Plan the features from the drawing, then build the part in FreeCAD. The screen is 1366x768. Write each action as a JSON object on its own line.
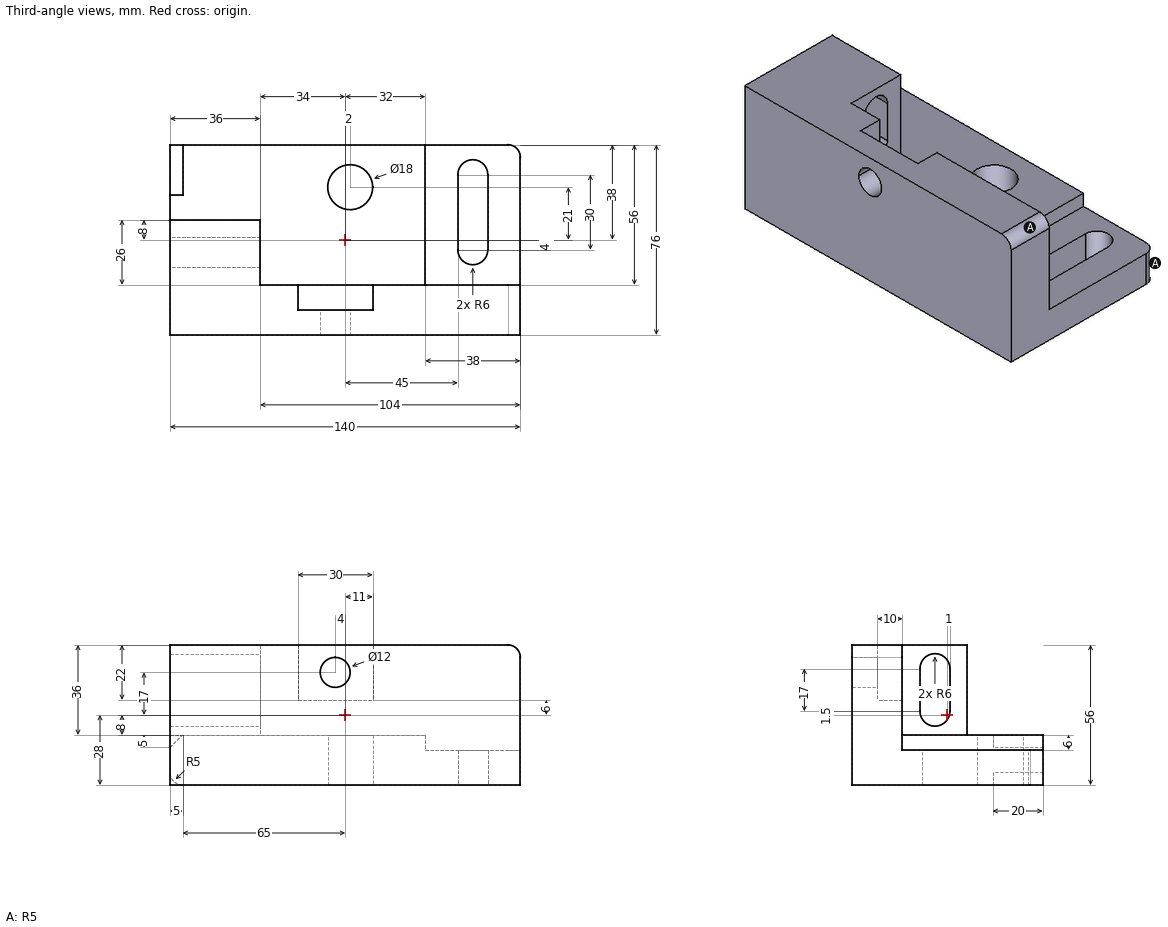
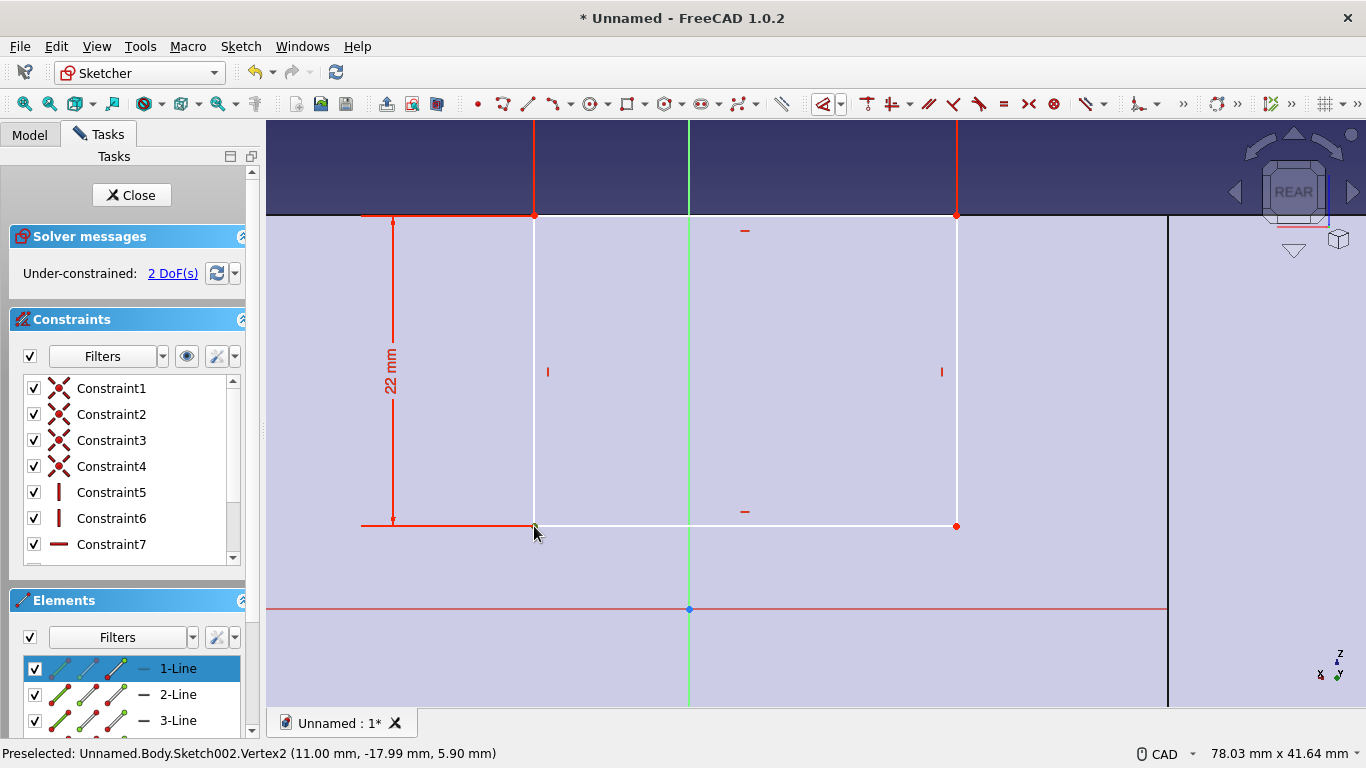
{"action": "key", "text": "i"}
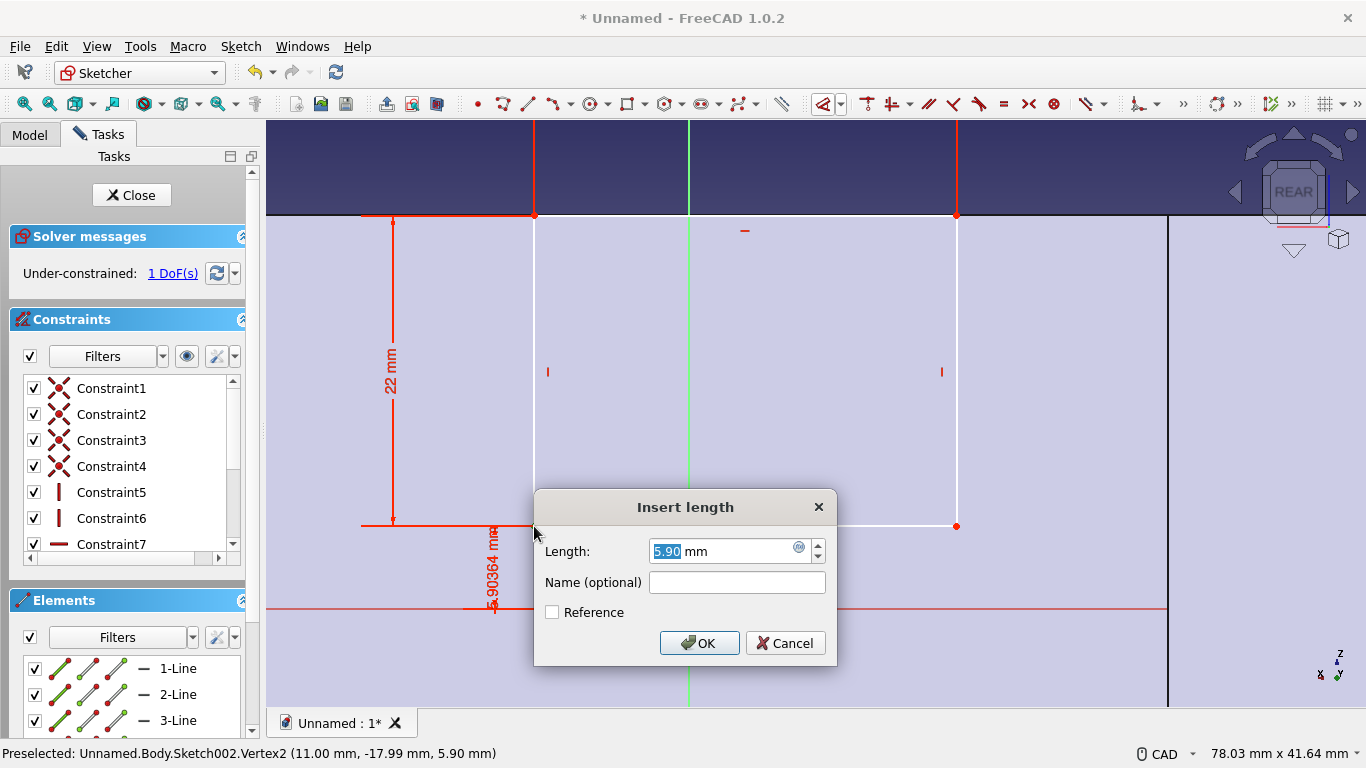
{"action": "type", "text": "6"}
{"action": "key", "text": "Return"}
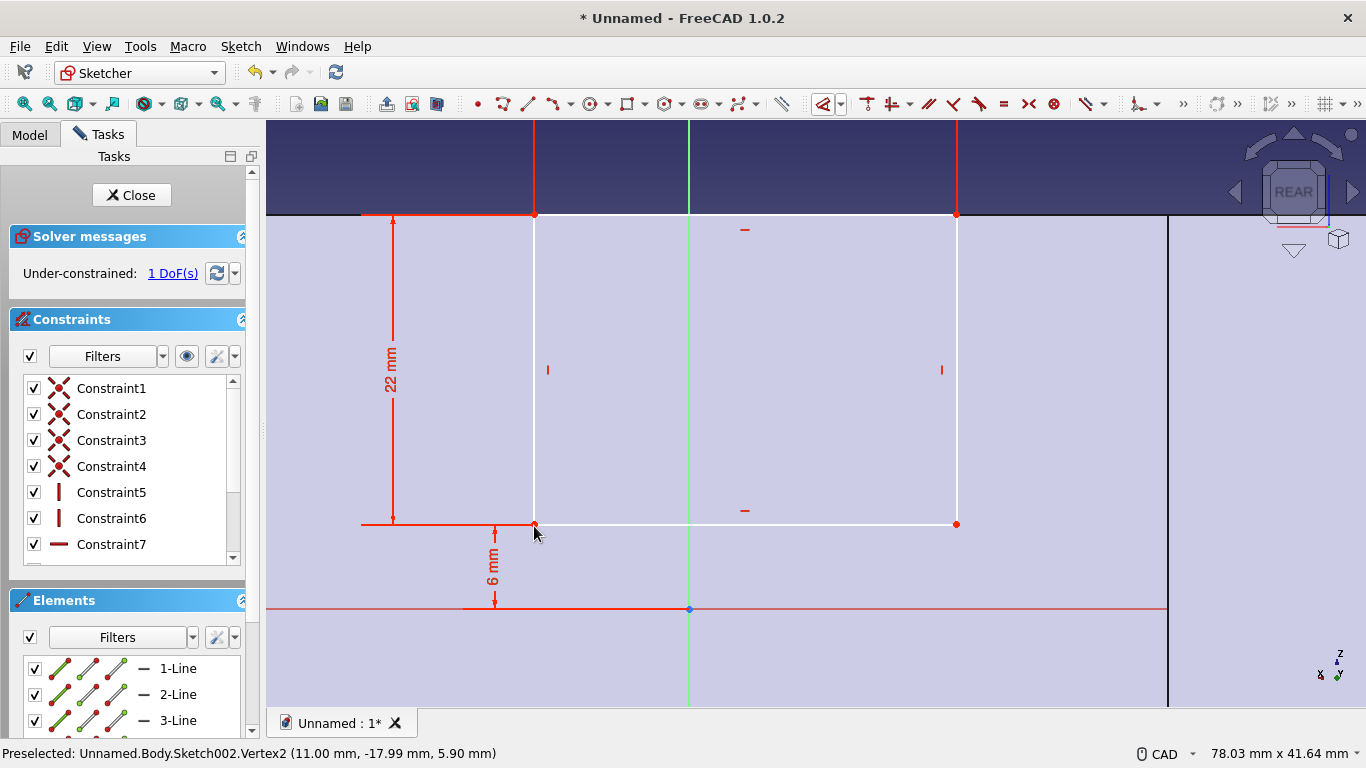
{"action": "left_click", "coordinate": [534, 215]}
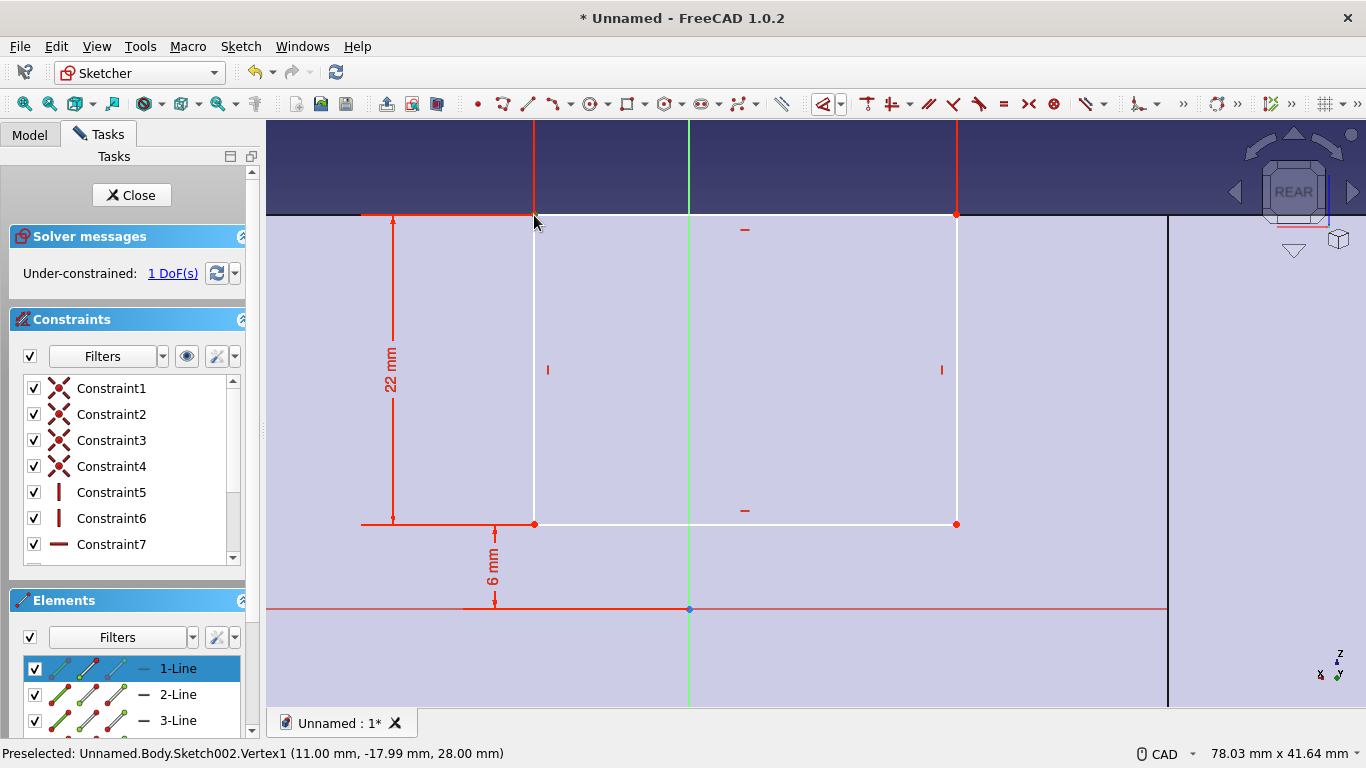
{"action": "key", "text": "l"}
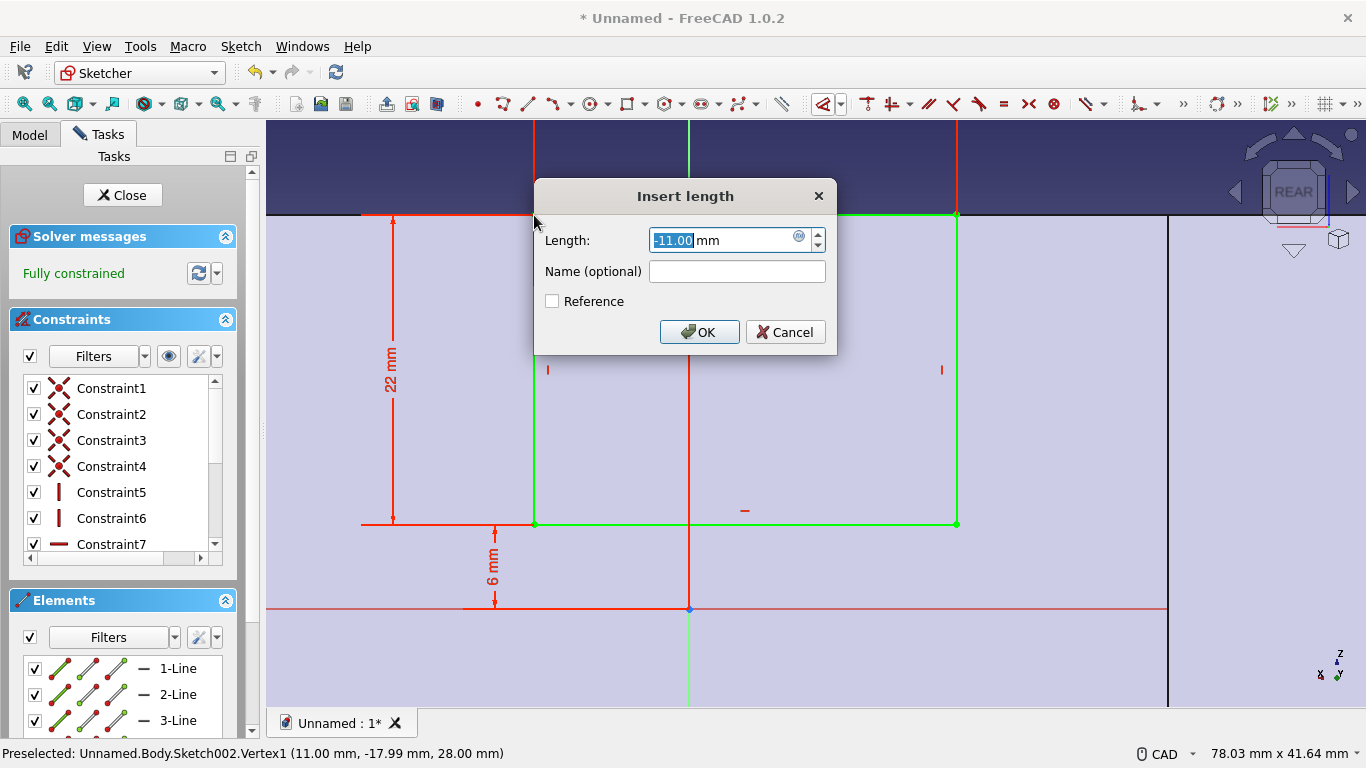
{"action": "type", "text": "-11"}
{"action": "key", "text": "Return"}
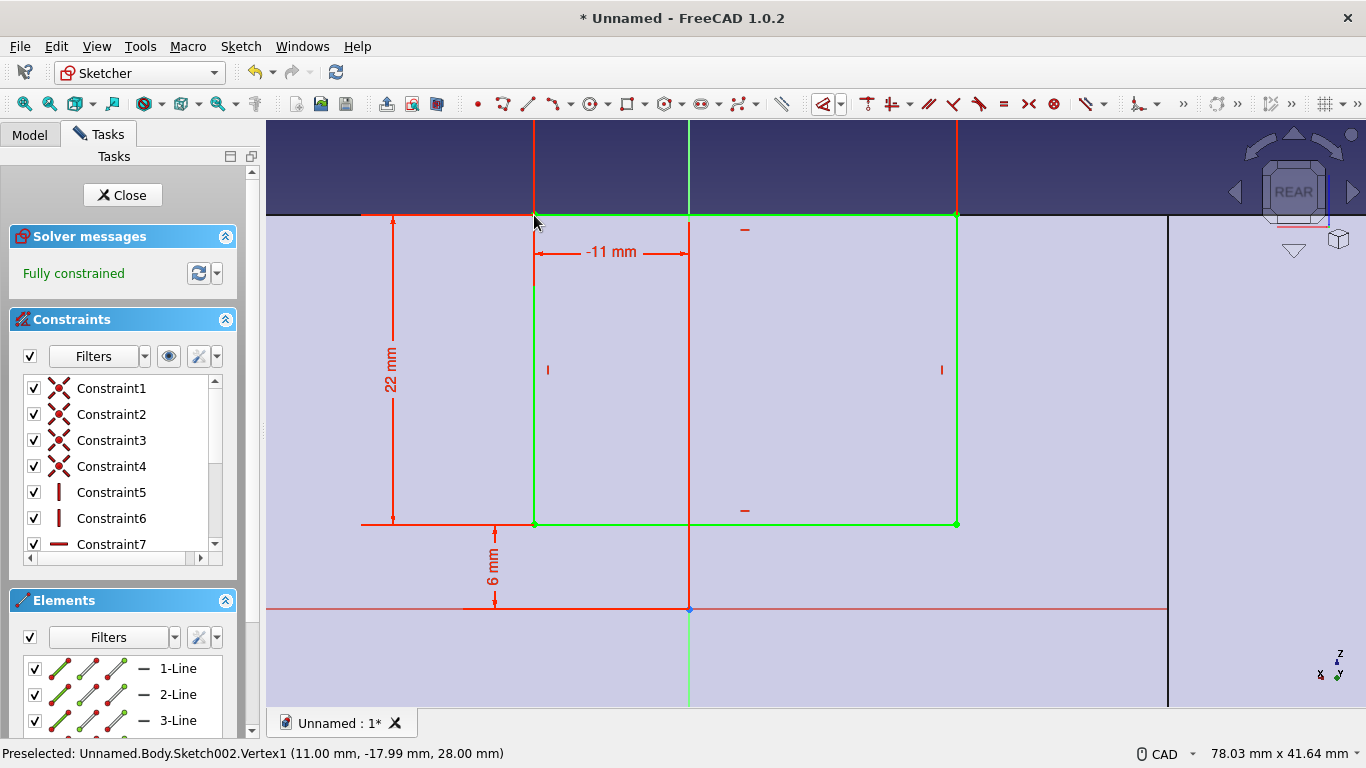
{"action": "left_click", "coordinate": [123, 195]}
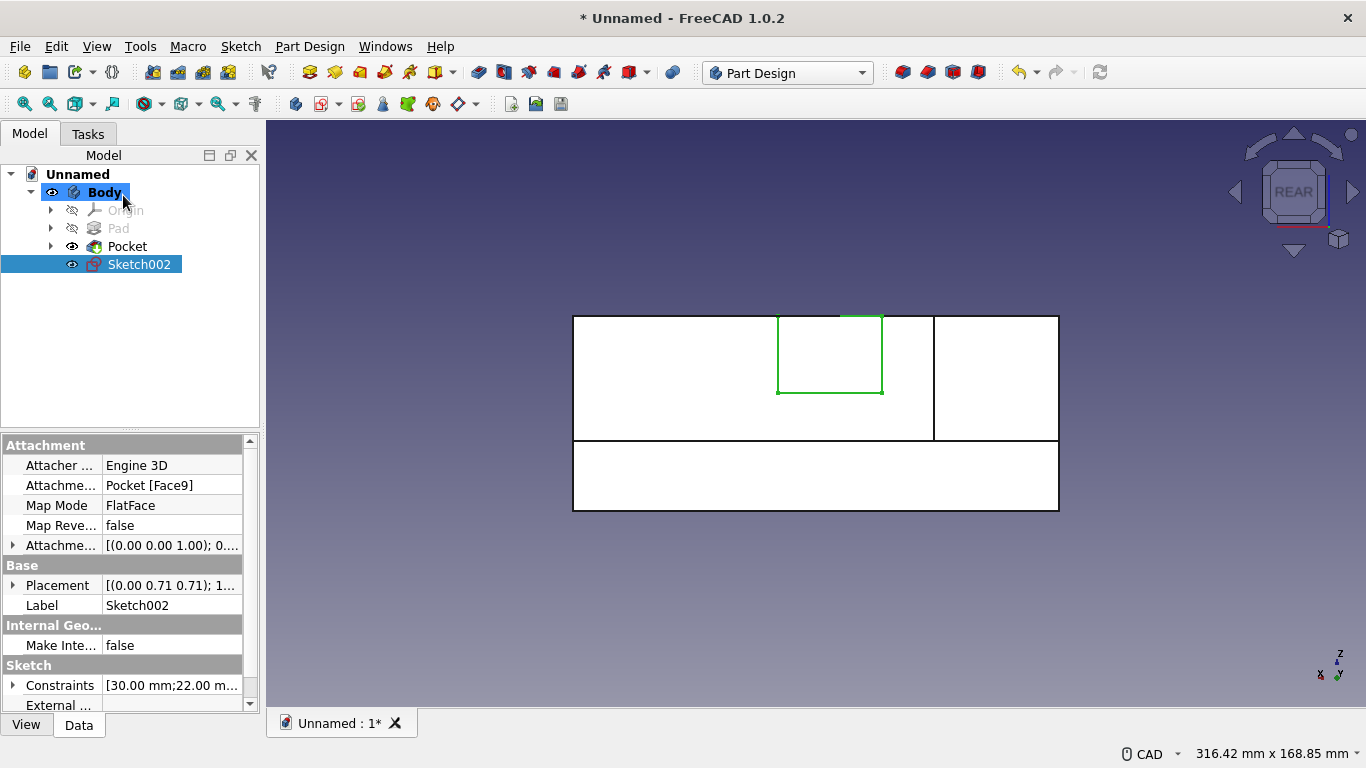
{"action": "left_click", "coordinate": [479, 72]}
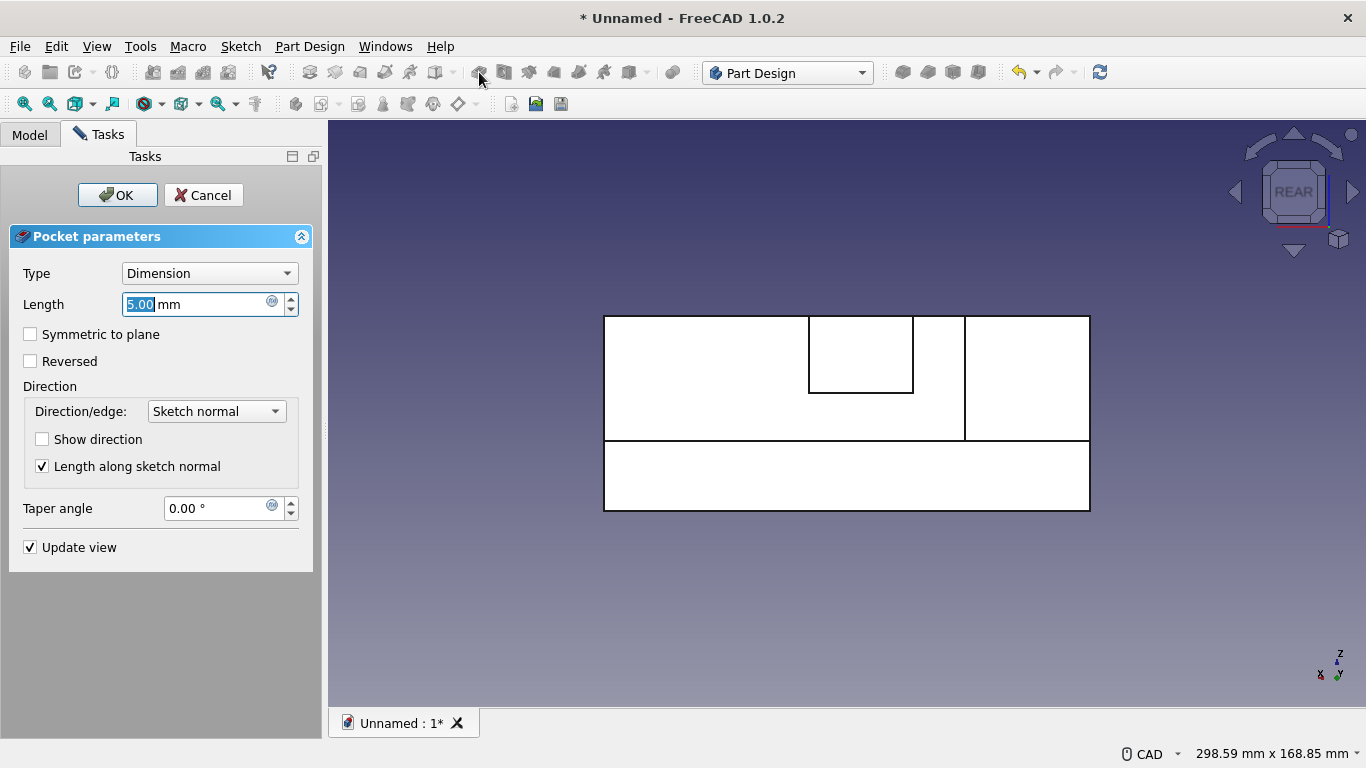
{"action": "type", "text": "10"}
{"action": "key", "text": "Tab"}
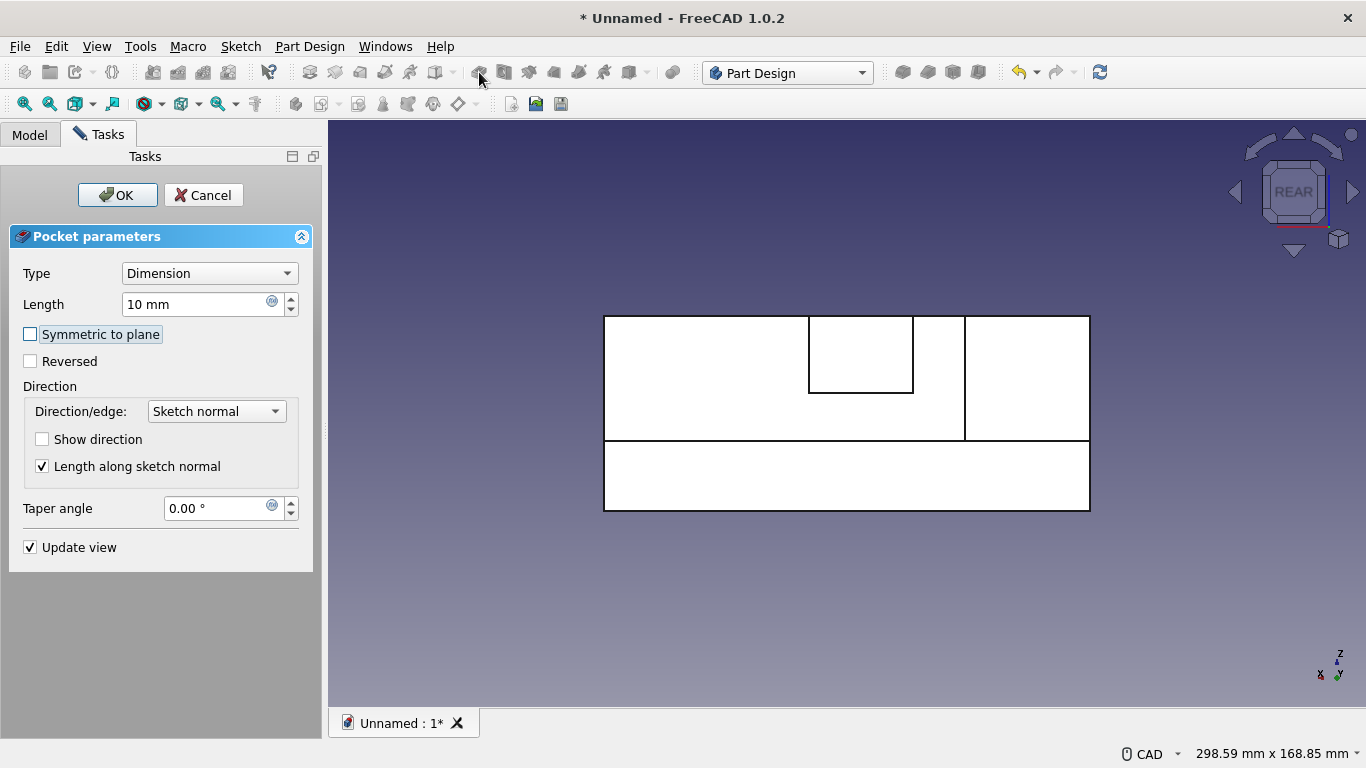
{"action": "left_click", "coordinate": [118, 195]}